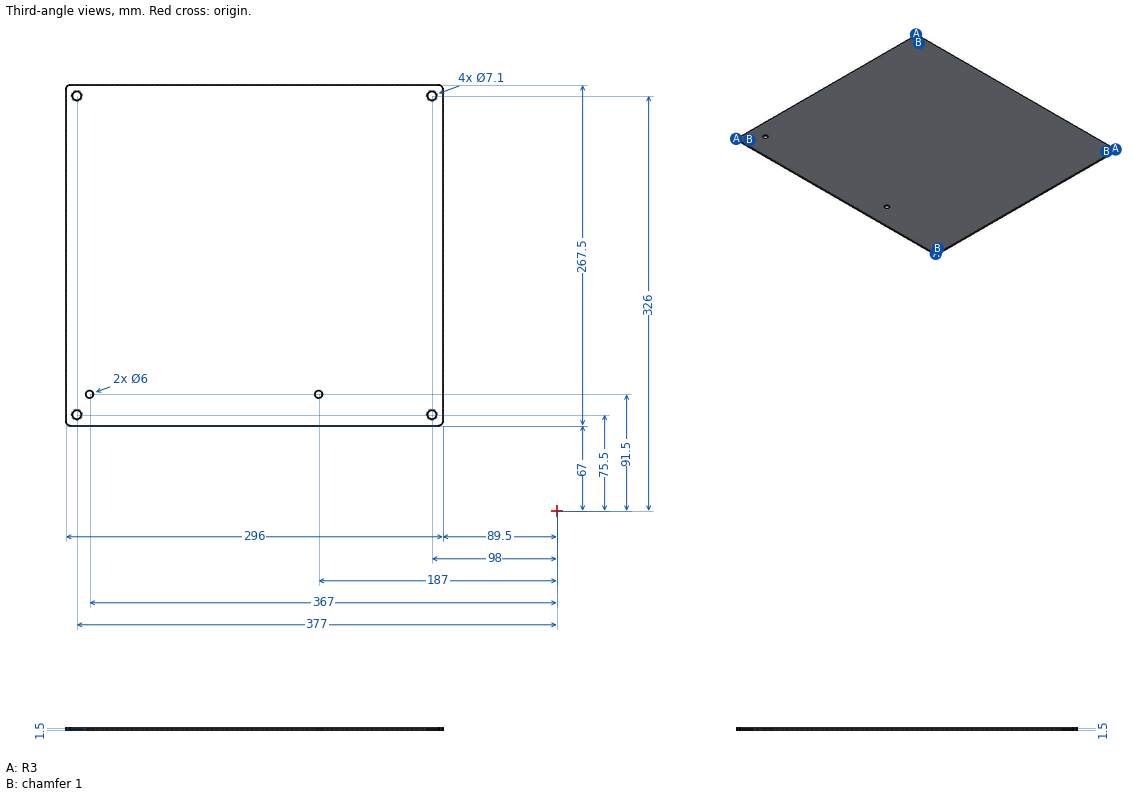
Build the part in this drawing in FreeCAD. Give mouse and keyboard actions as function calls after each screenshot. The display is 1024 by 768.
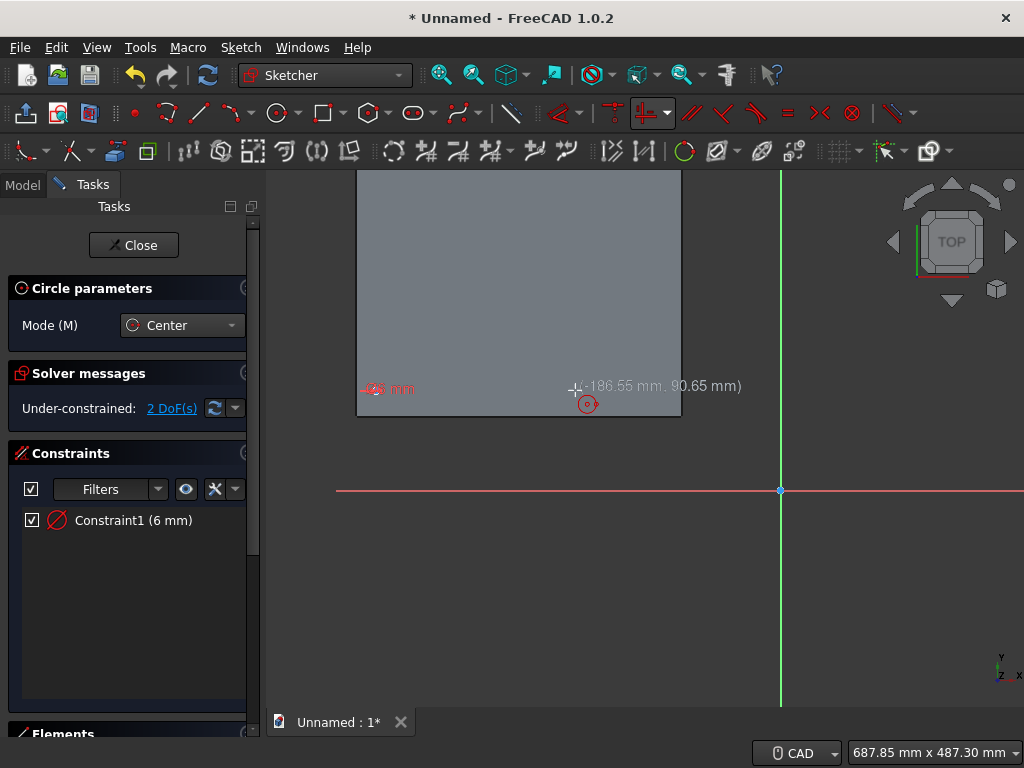
click(575, 390)
move(577, 388)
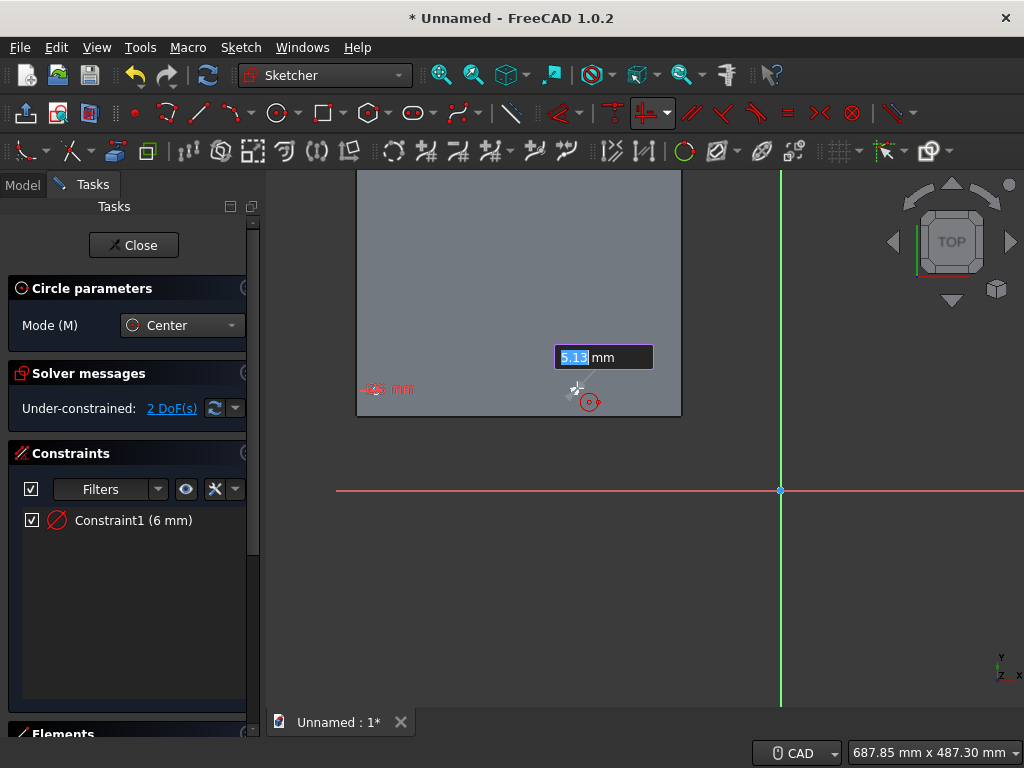
text(6)
key(Return)
key(Escape)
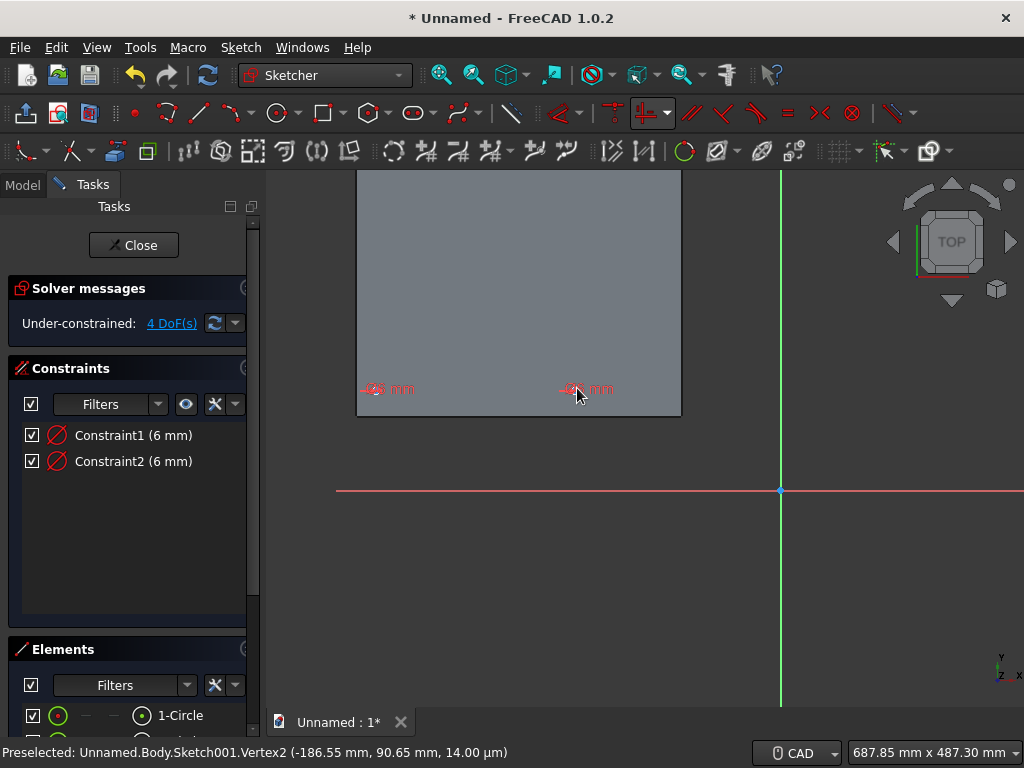
click(376, 391)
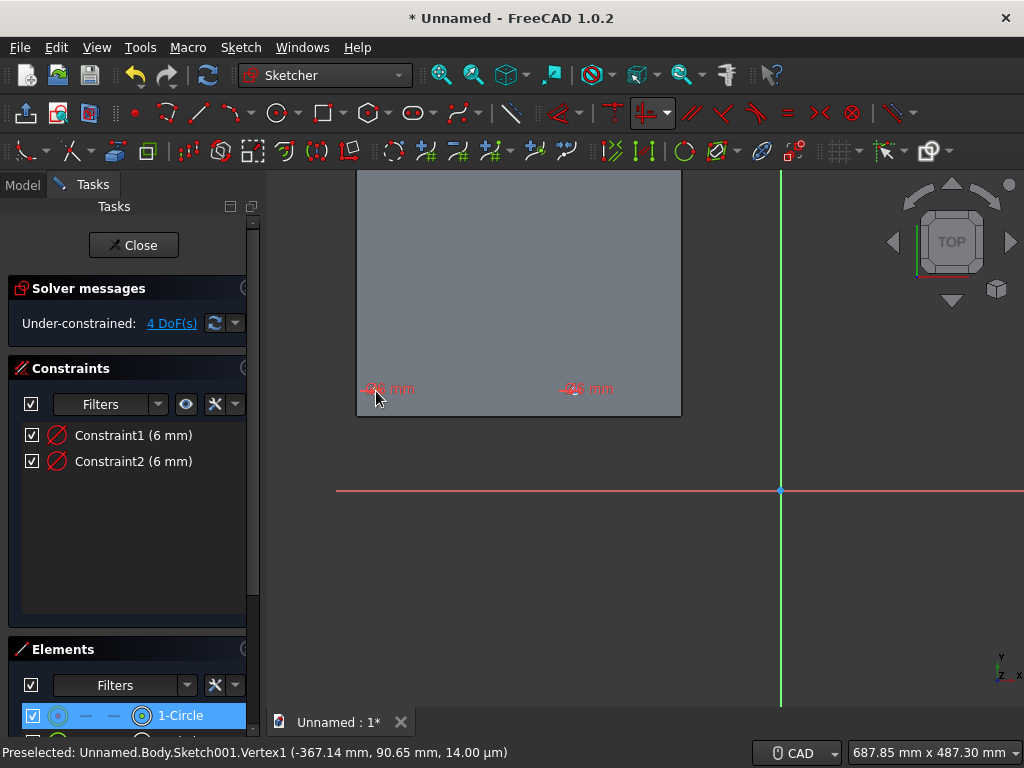
click(575, 391)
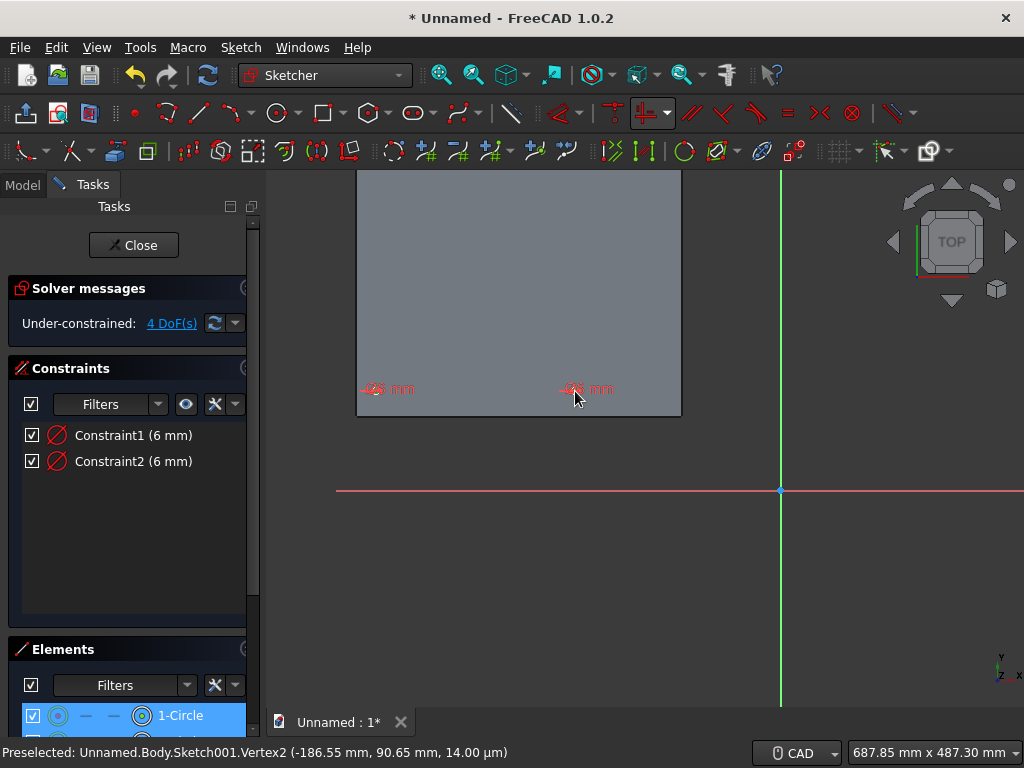
key(h)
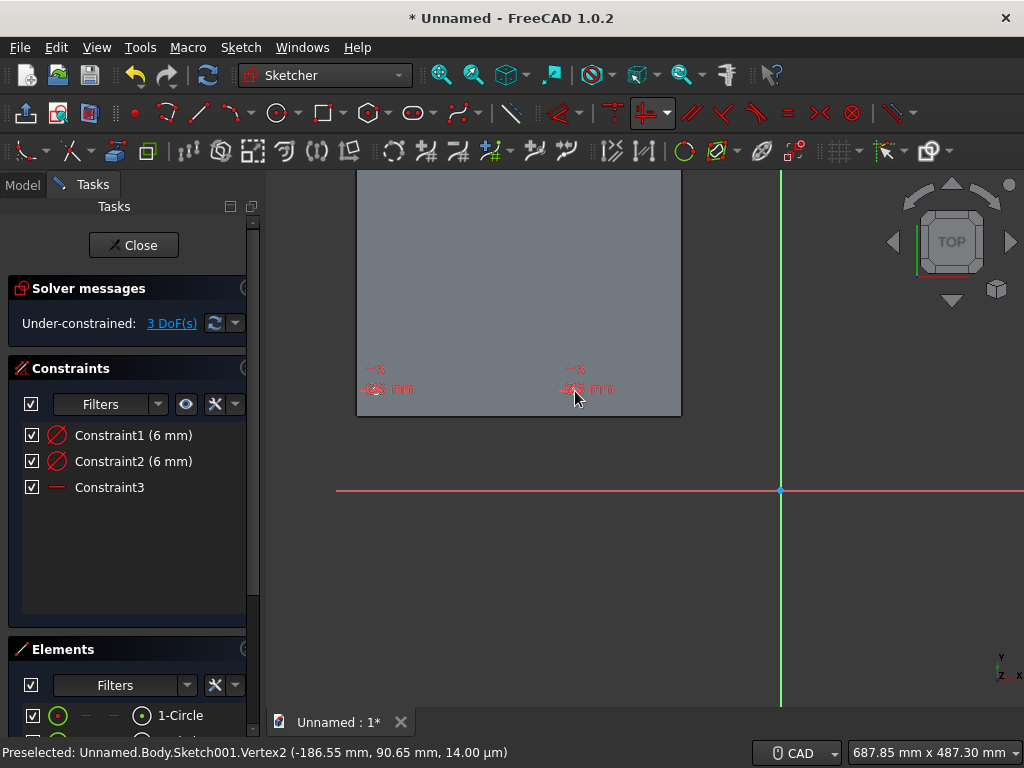
click(558, 114)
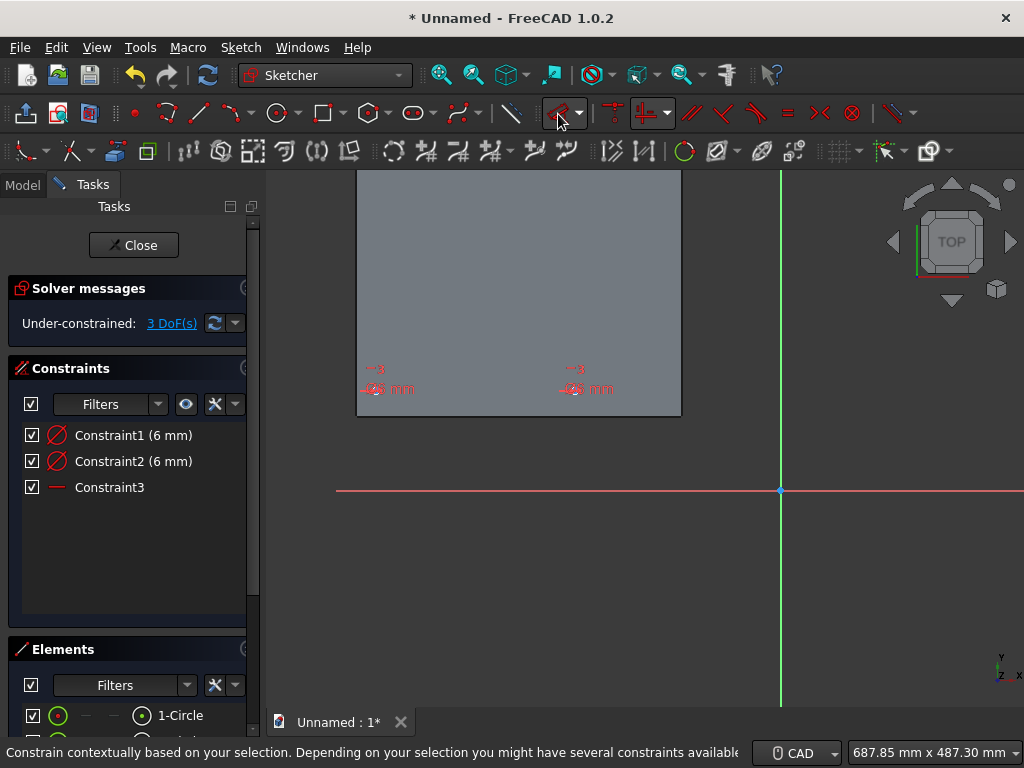
click(376, 391)
click(578, 525)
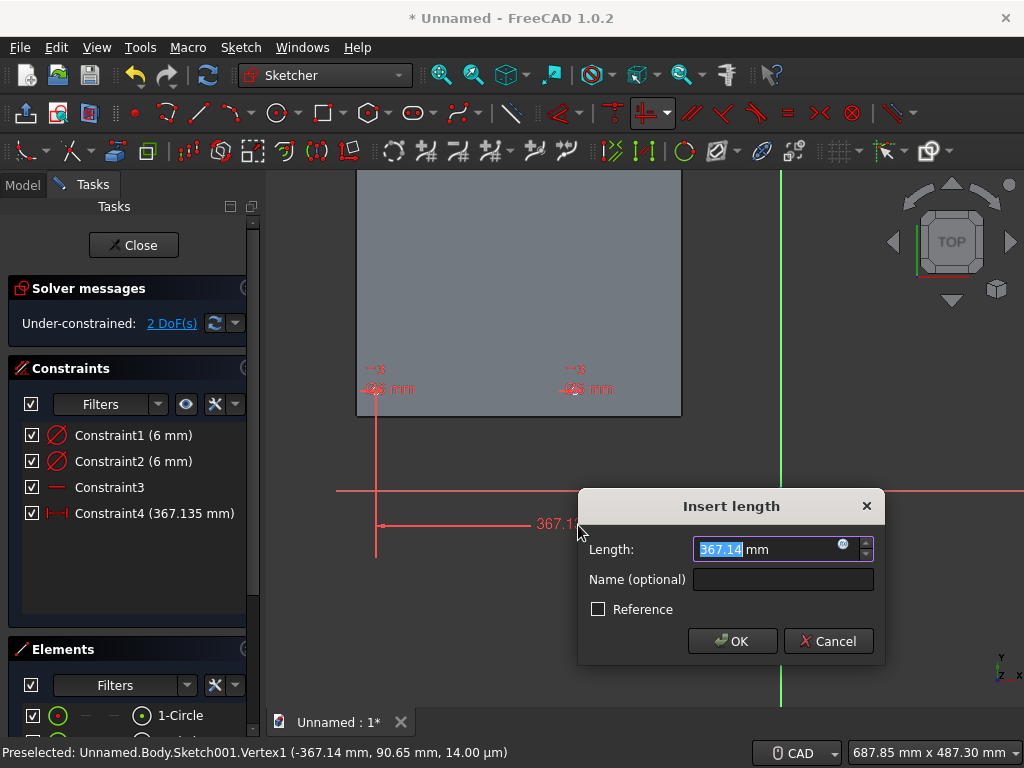
text(367)
key(Return)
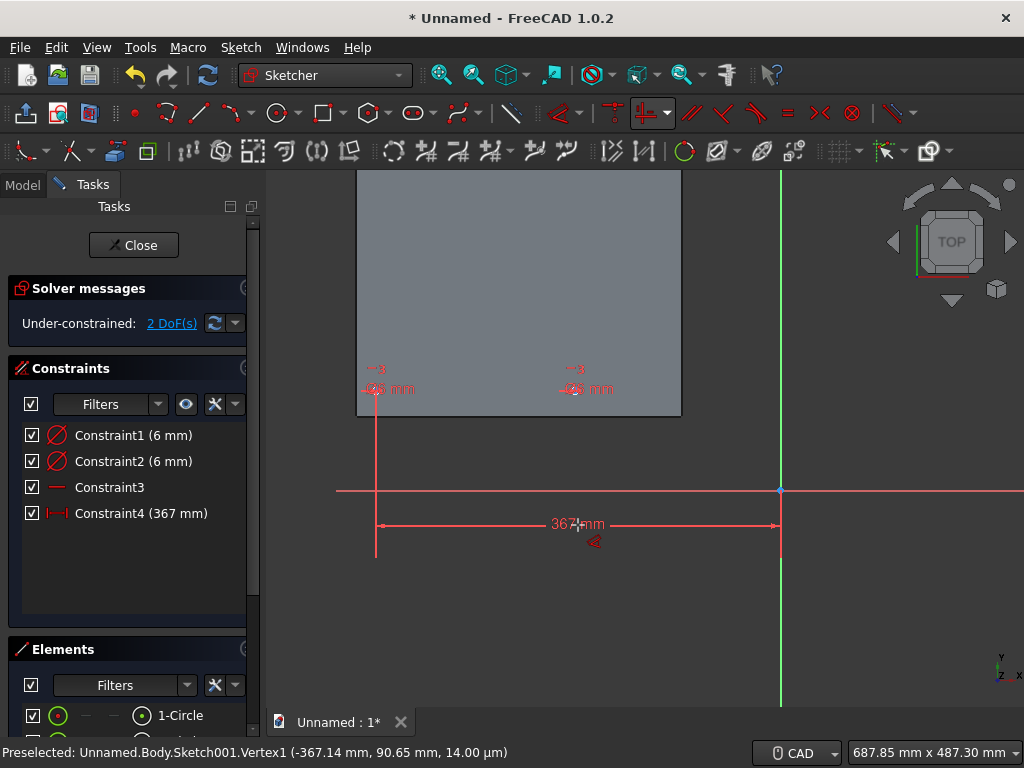
click(575, 391)
click(678, 525)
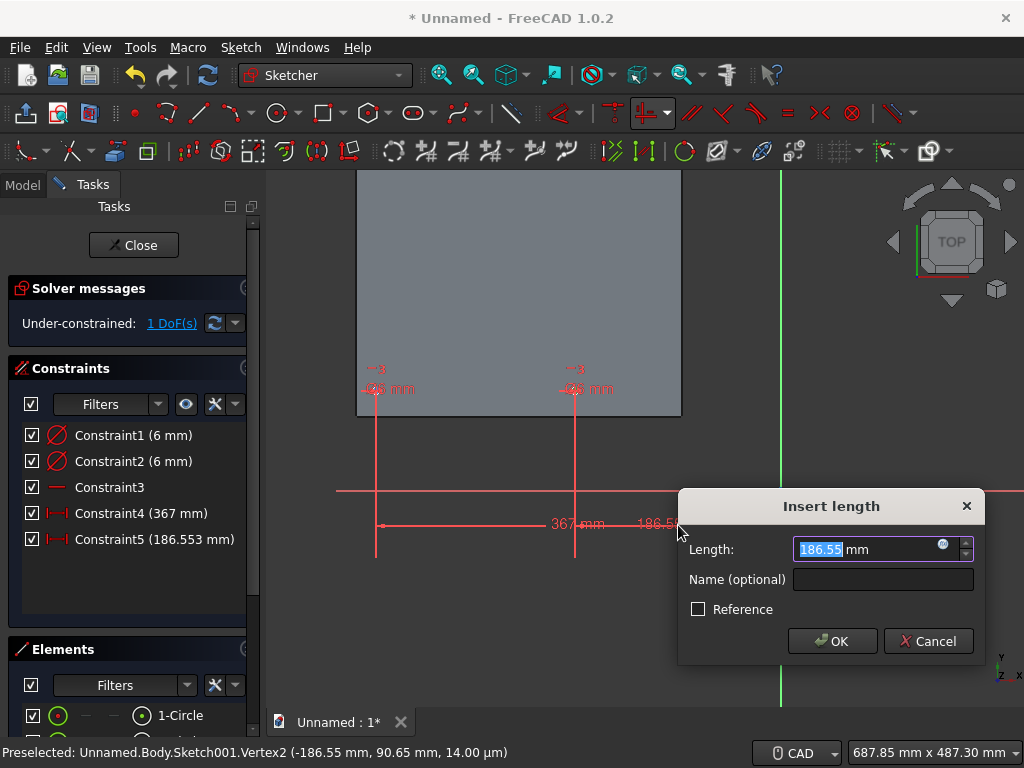
text(187)
key(Return)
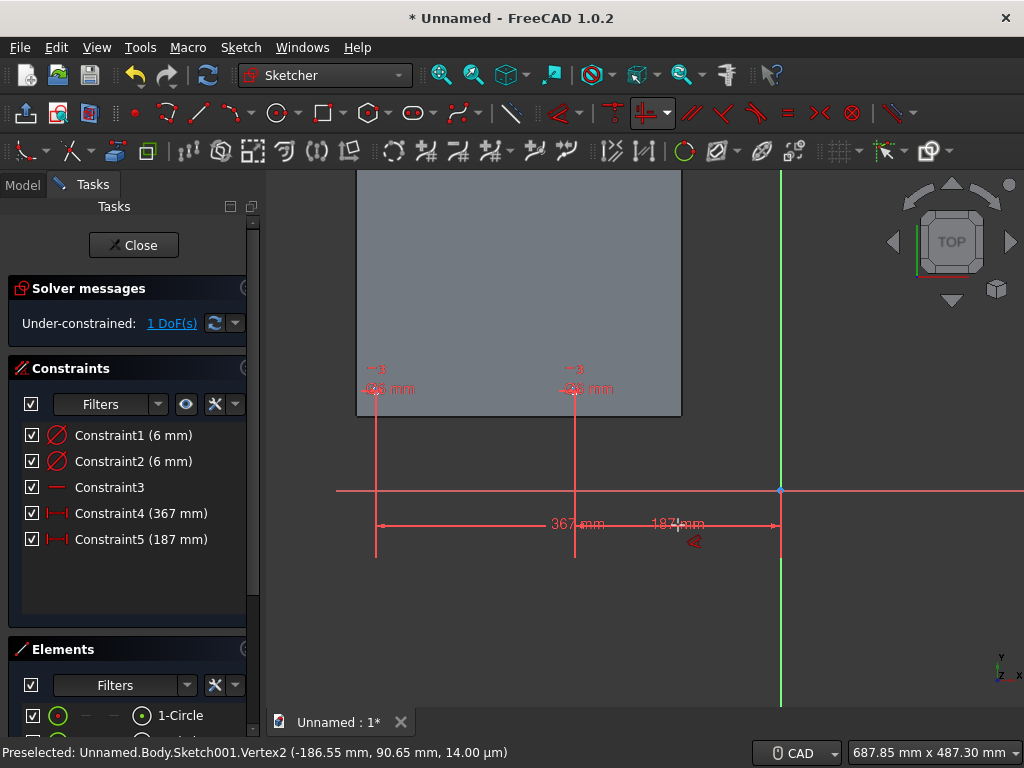
click(376, 391)
click(815, 441)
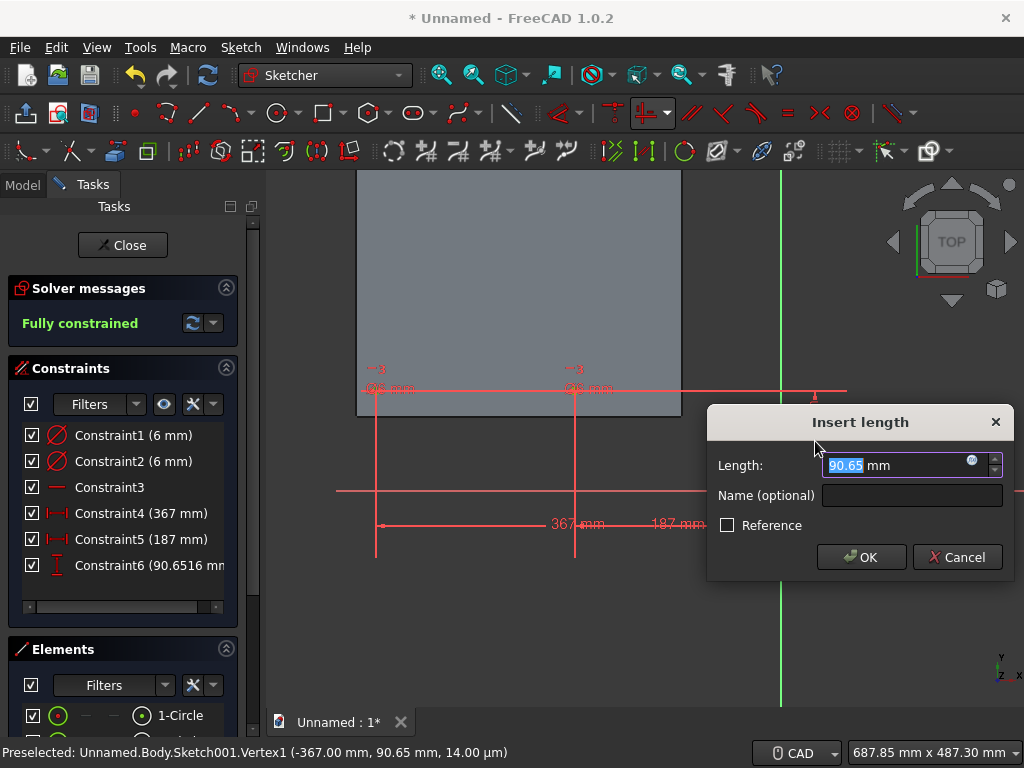
text(91.5)
key(Return)
key(Escape)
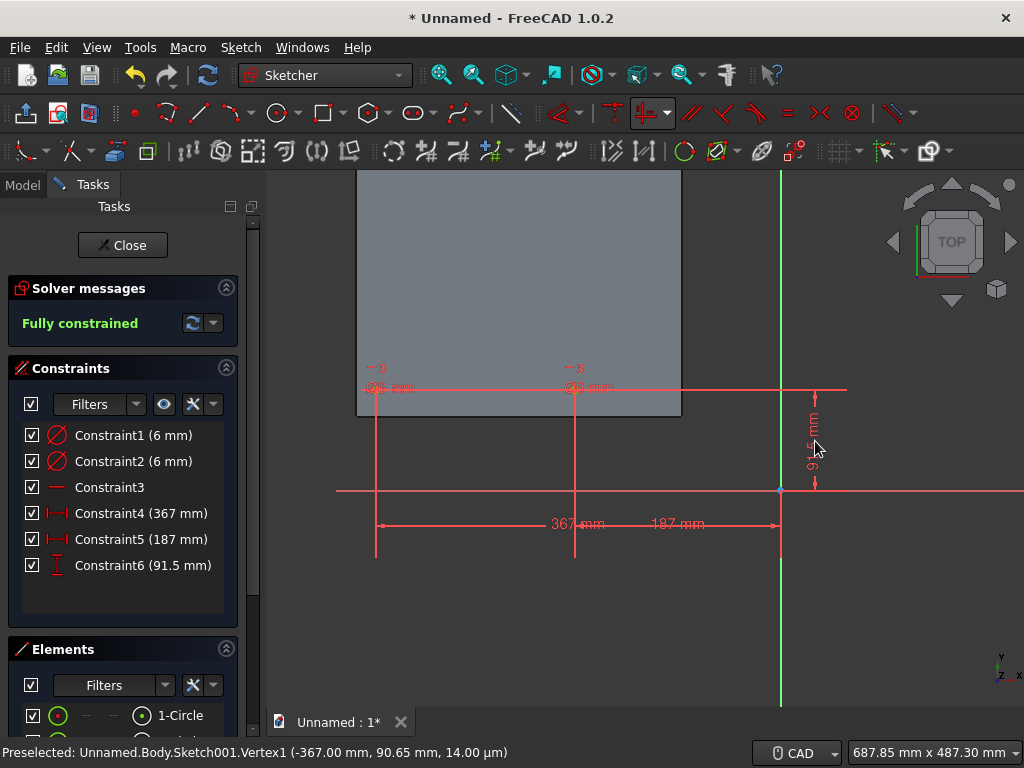
click(123, 245)